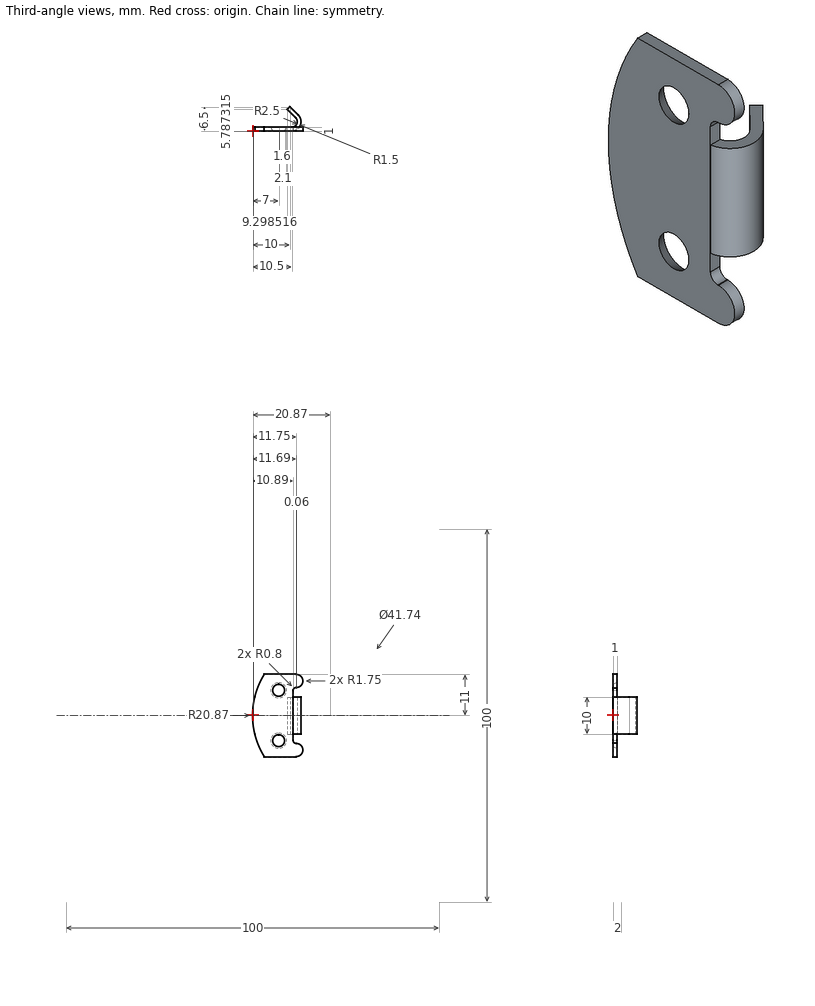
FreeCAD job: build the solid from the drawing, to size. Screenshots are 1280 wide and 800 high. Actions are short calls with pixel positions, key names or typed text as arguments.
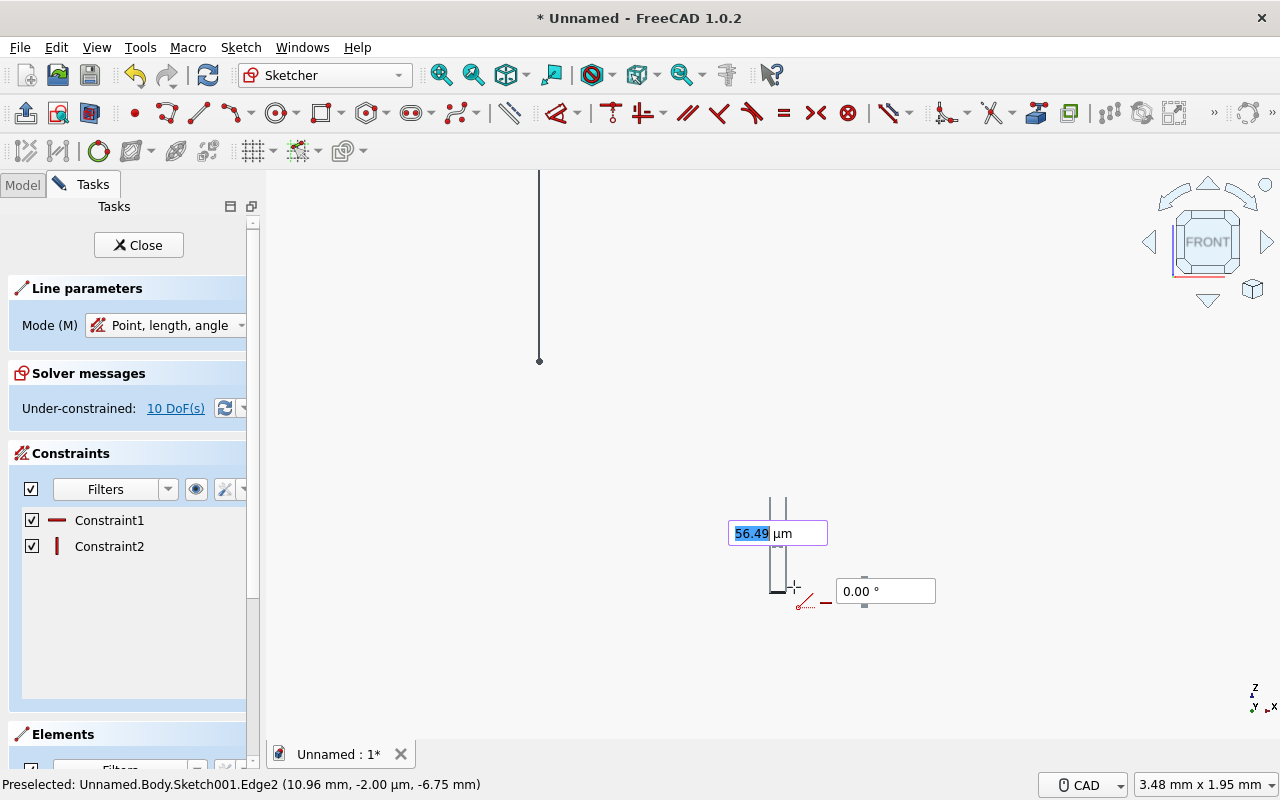
click(785, 576)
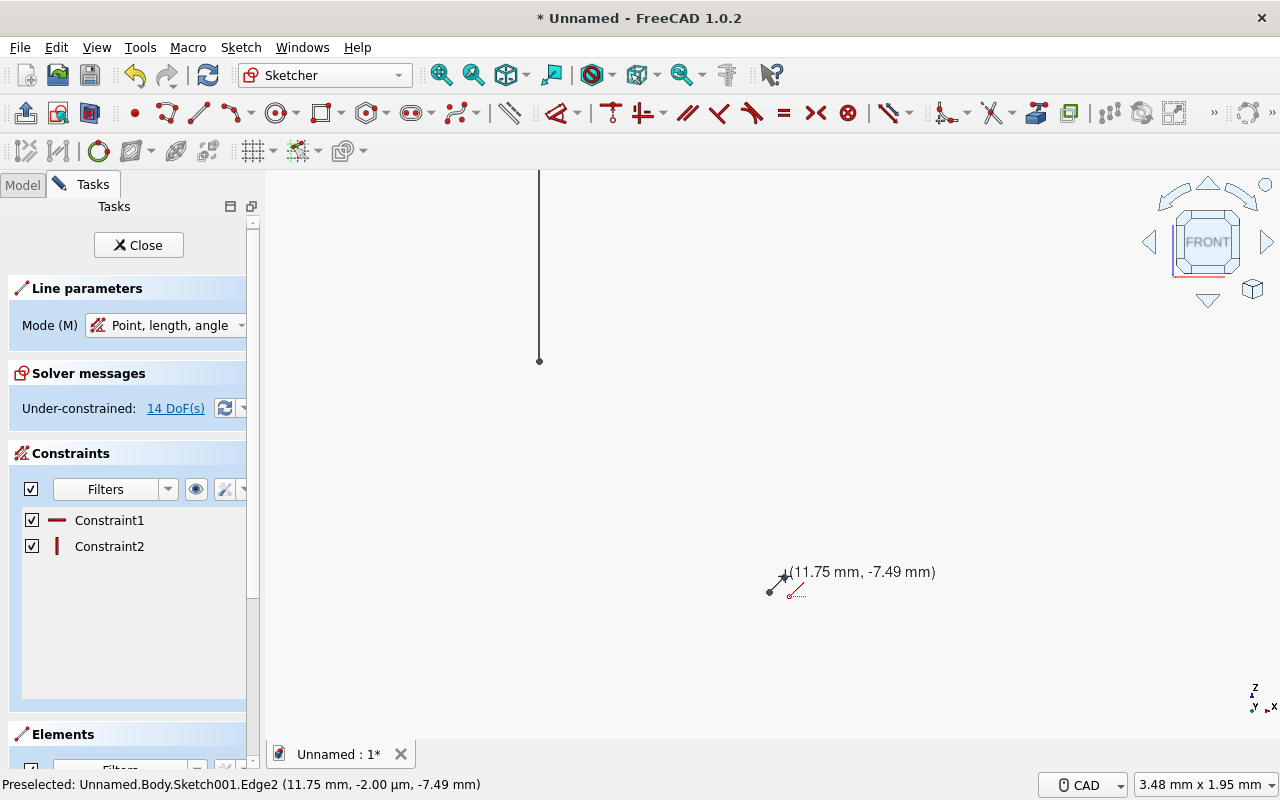
scroll(794, 588, down, 14)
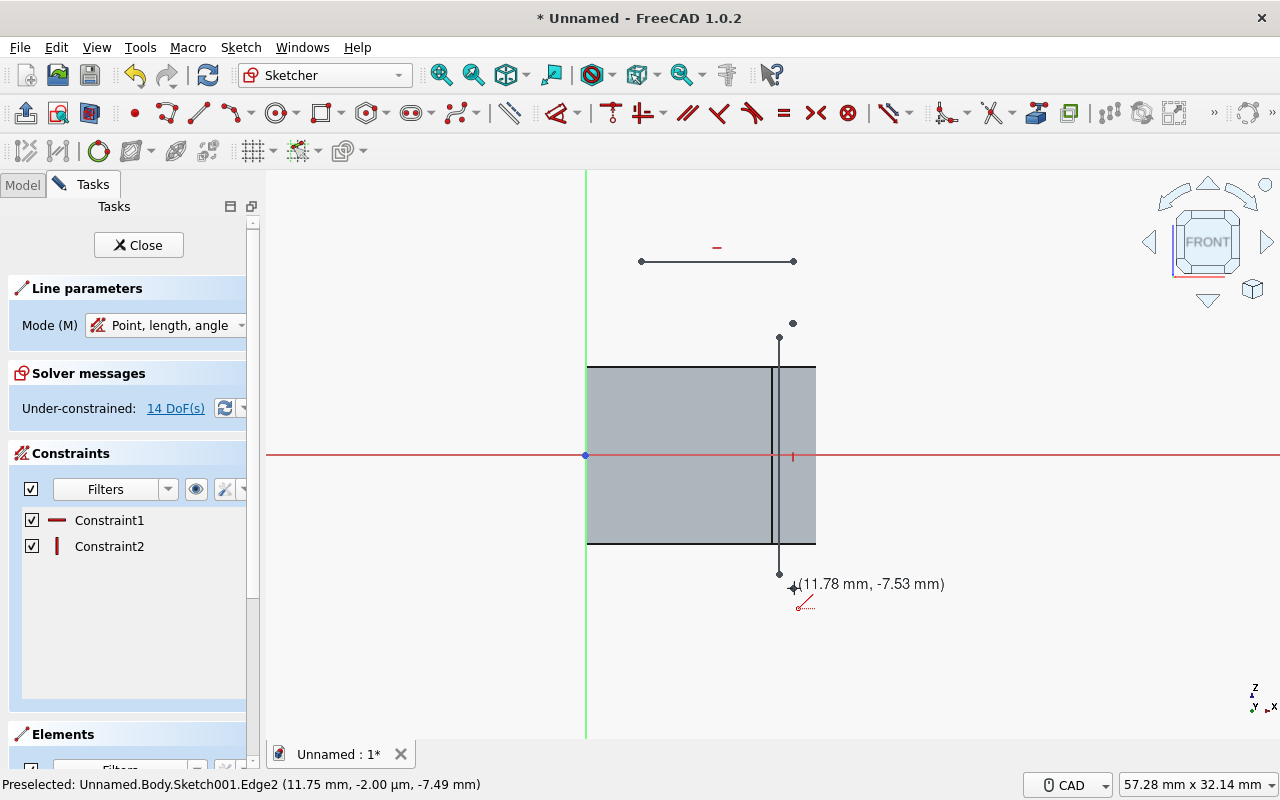
click(794, 650)
click(641, 650)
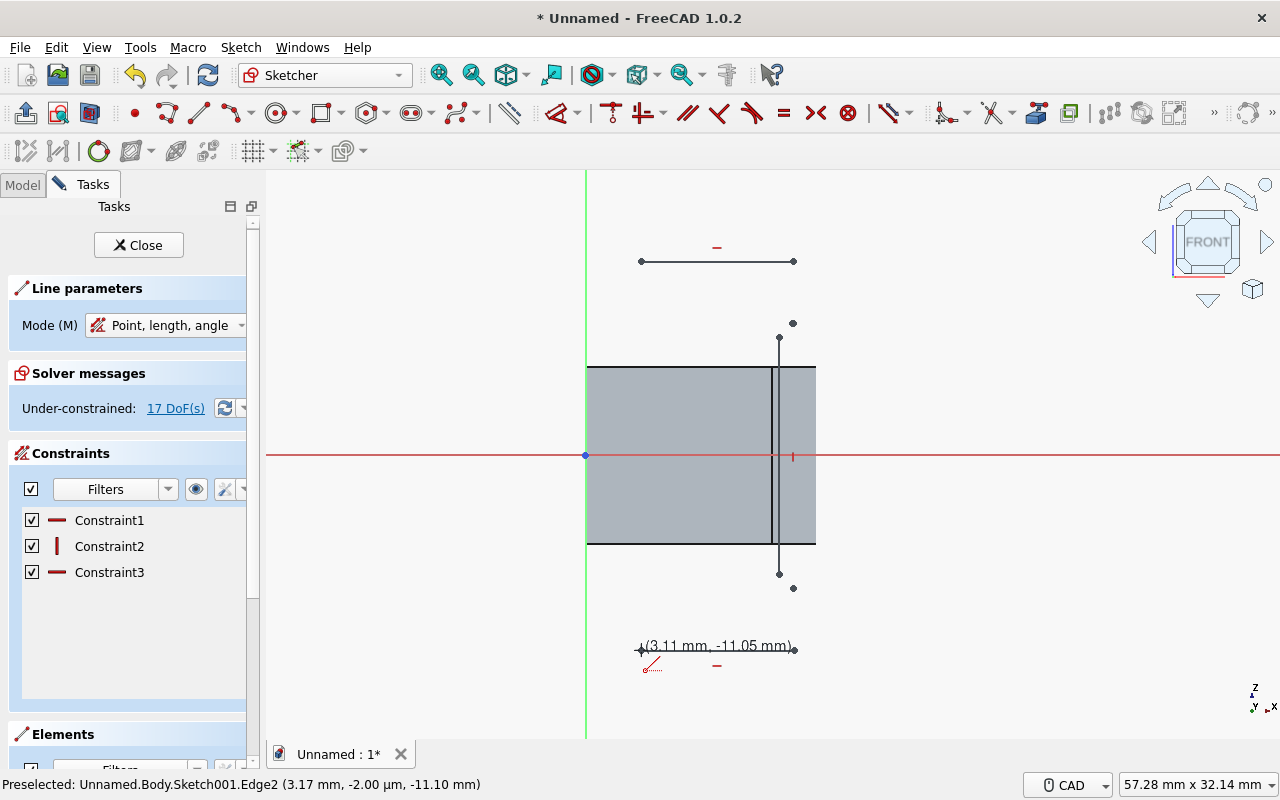
click(232, 114)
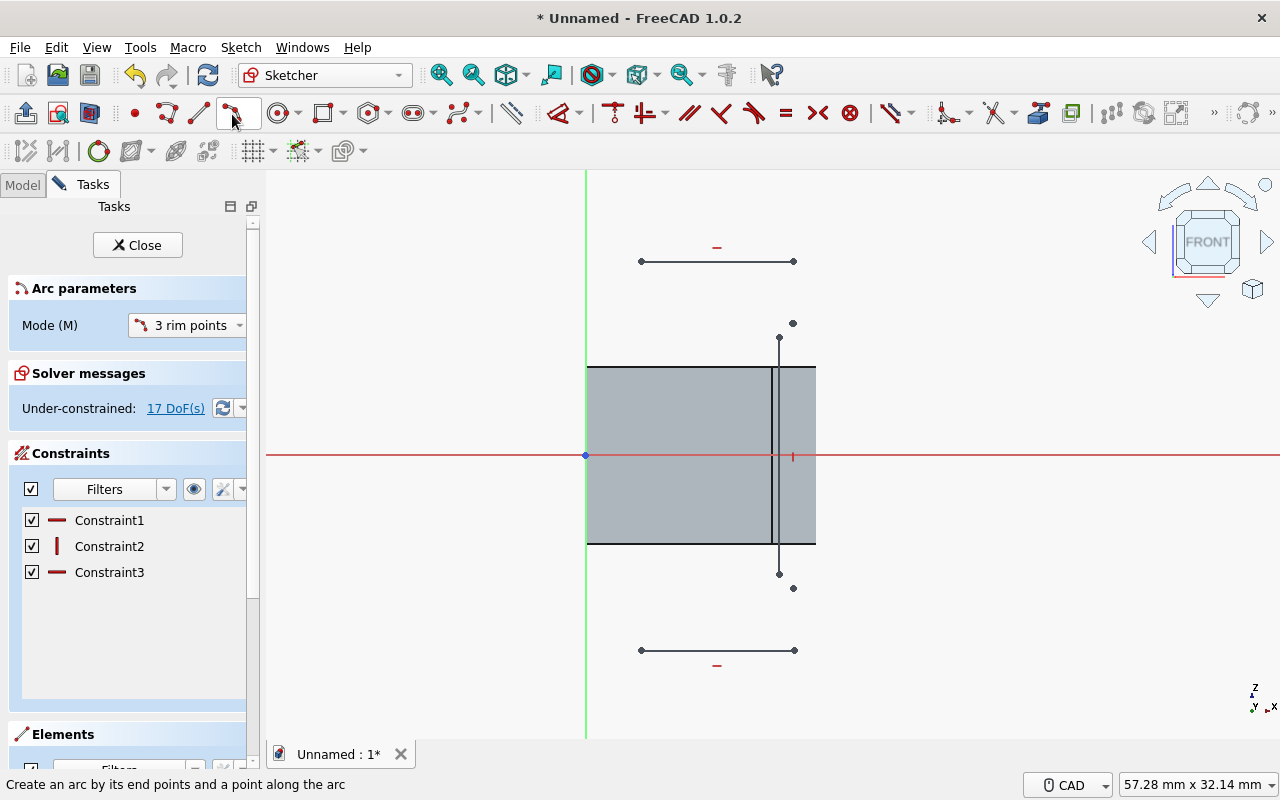
click(794, 262)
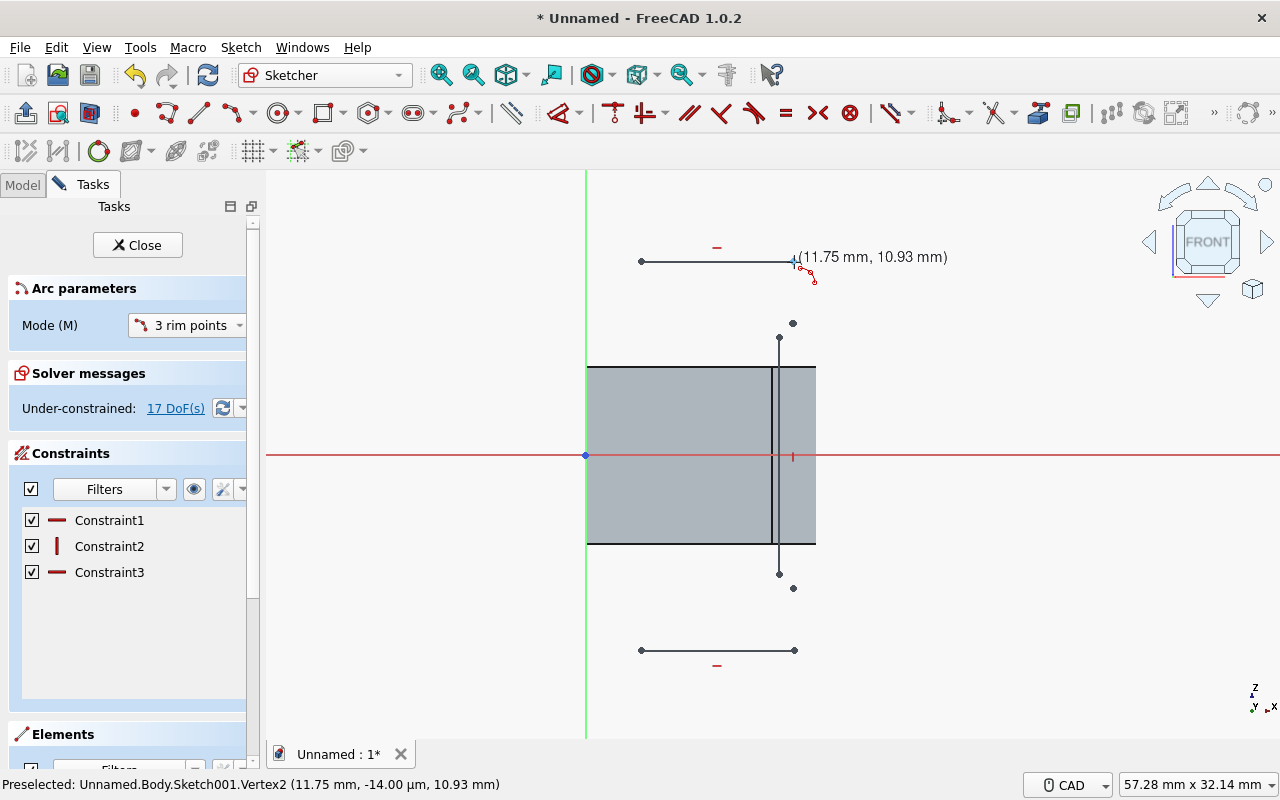
scroll(794, 323, up, 17)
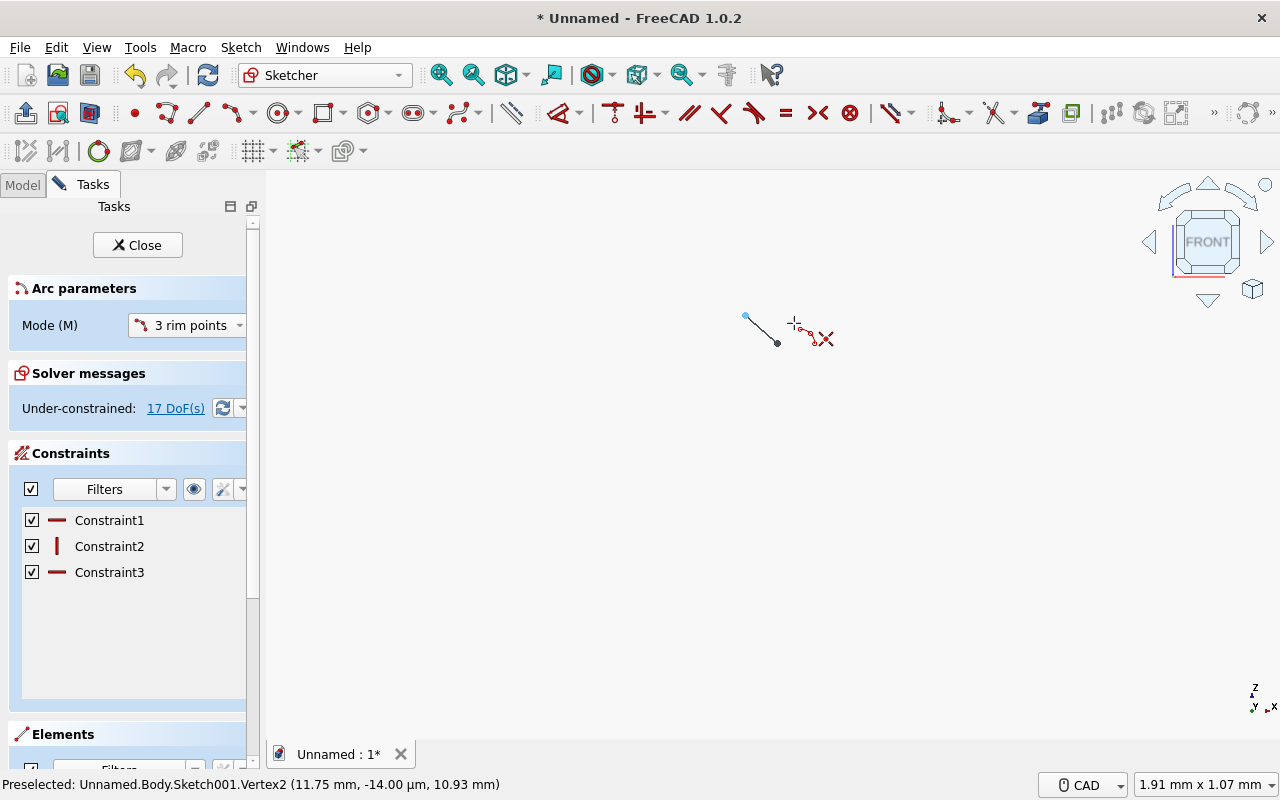
click(777, 313)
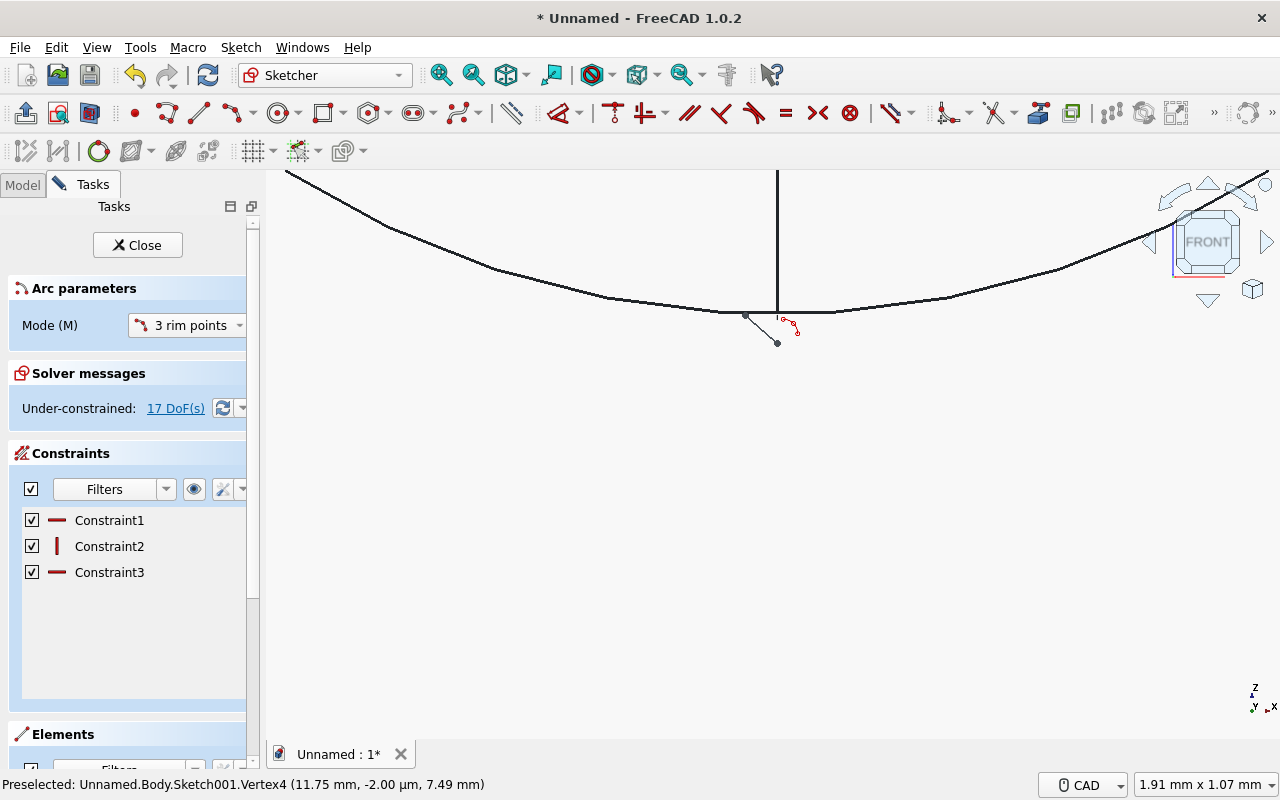
scroll(794, 322, down, 17)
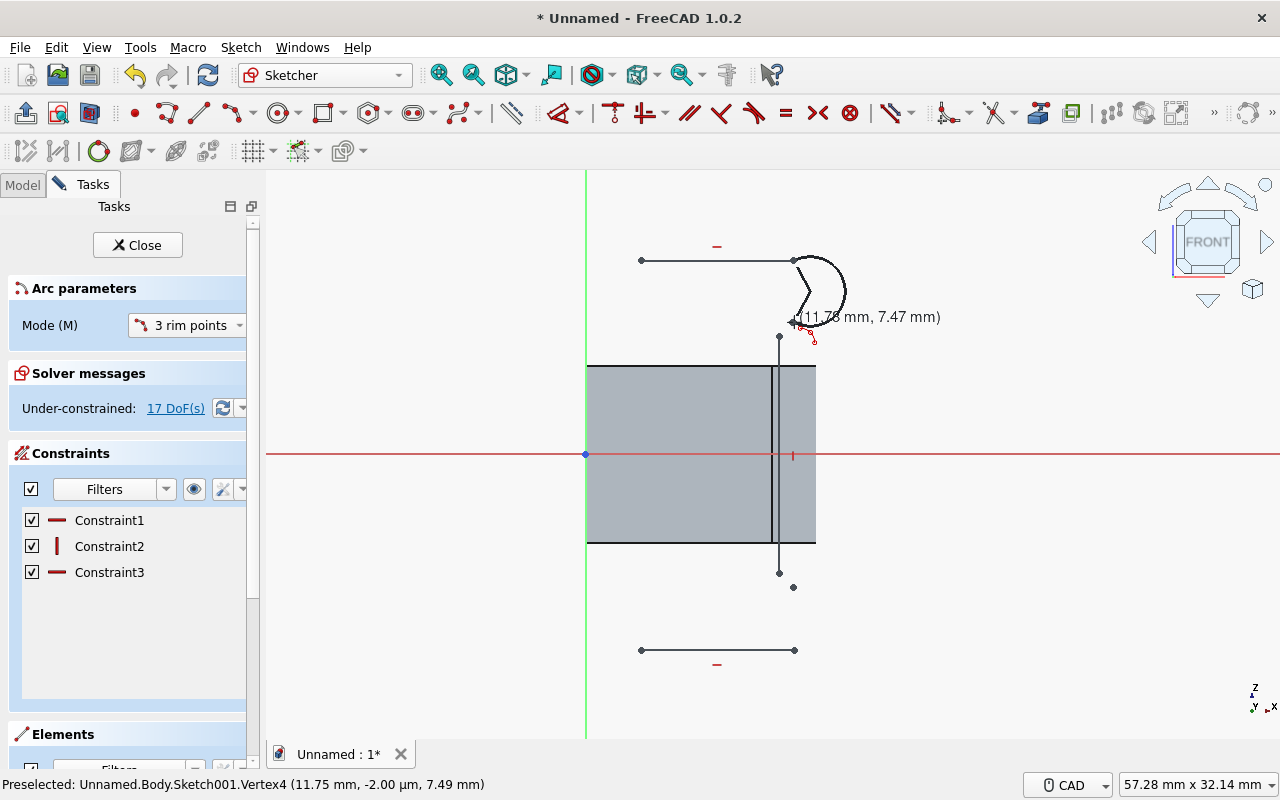
click(825, 291)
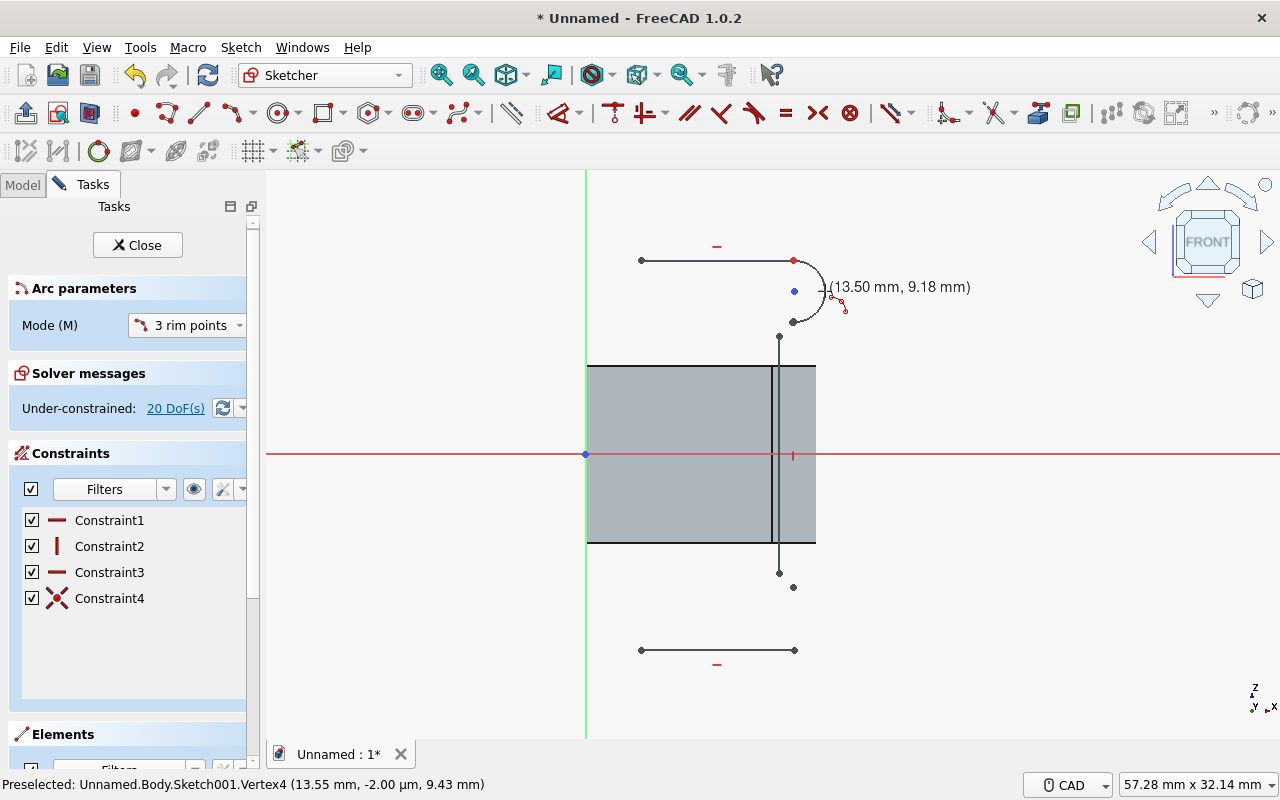
scroll(793, 322, up, 17)